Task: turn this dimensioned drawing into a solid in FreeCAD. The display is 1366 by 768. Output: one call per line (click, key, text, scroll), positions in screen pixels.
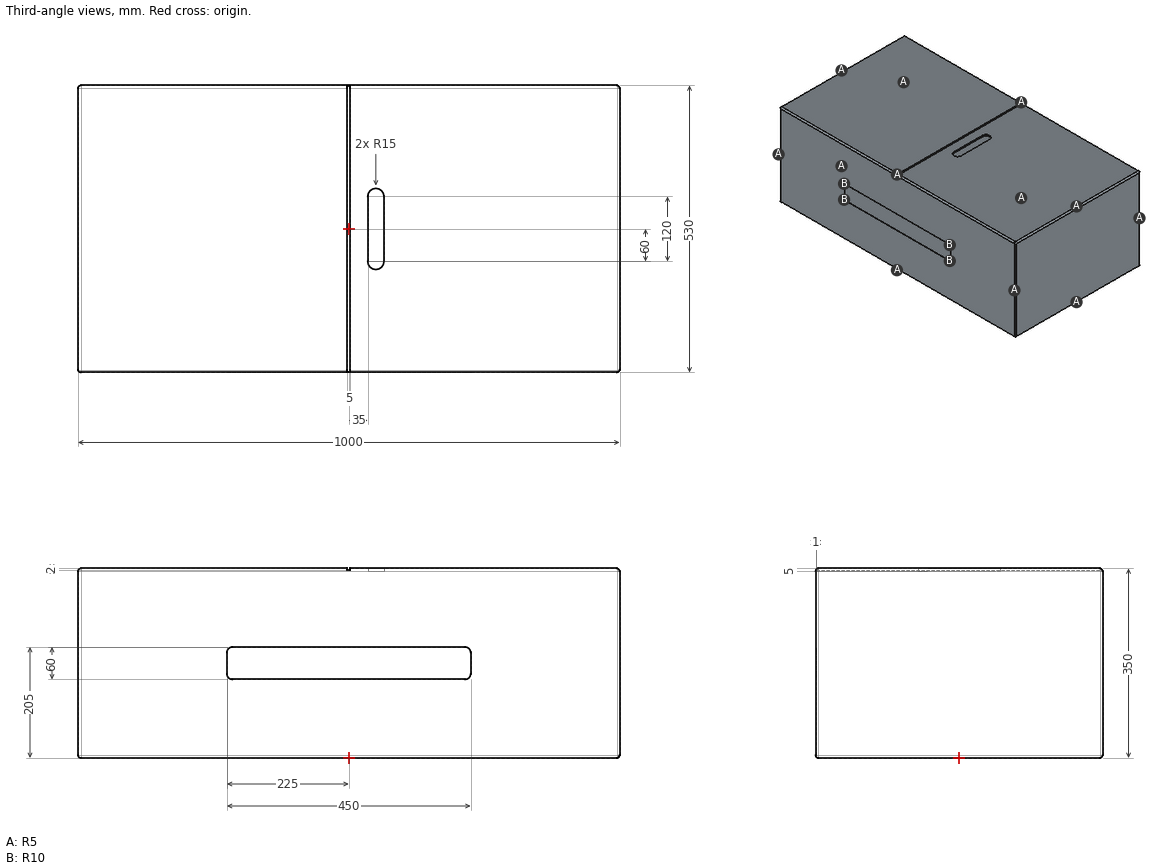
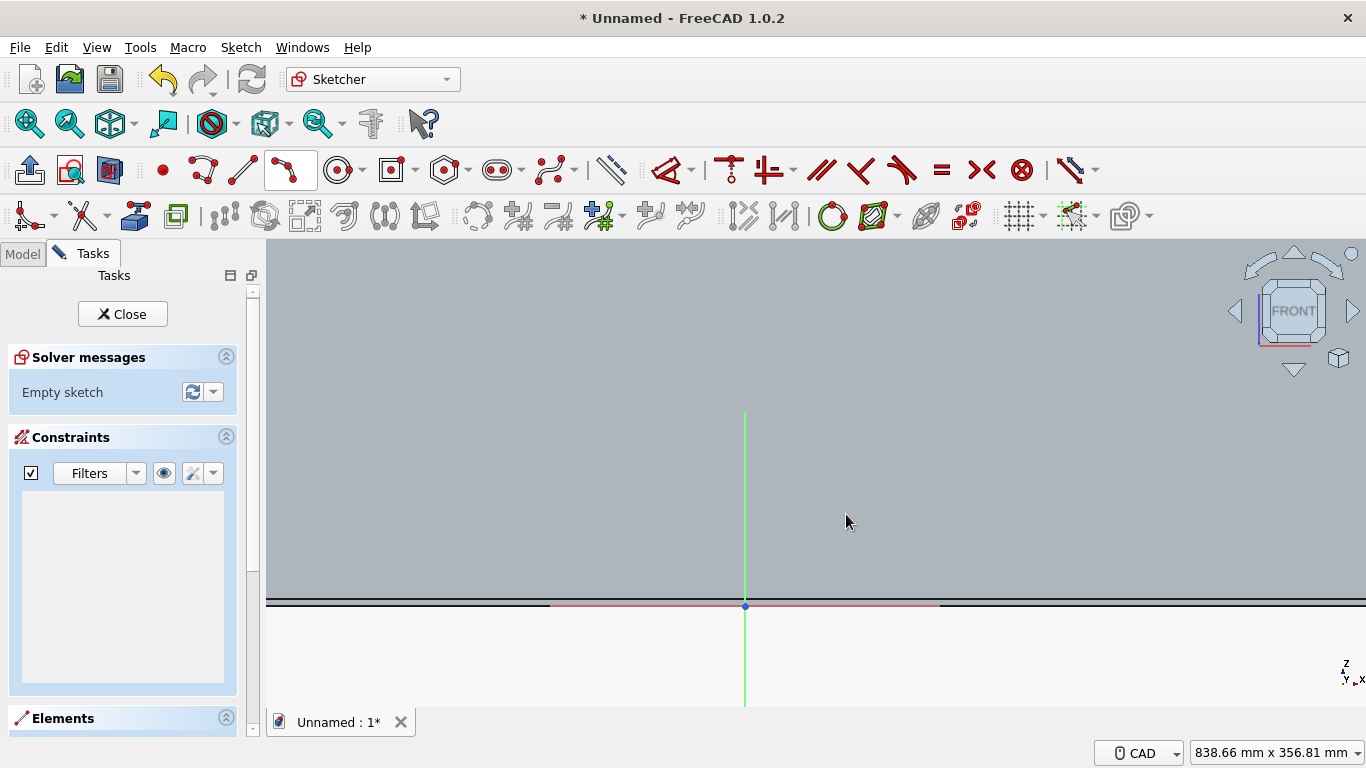
key(g)
key(r)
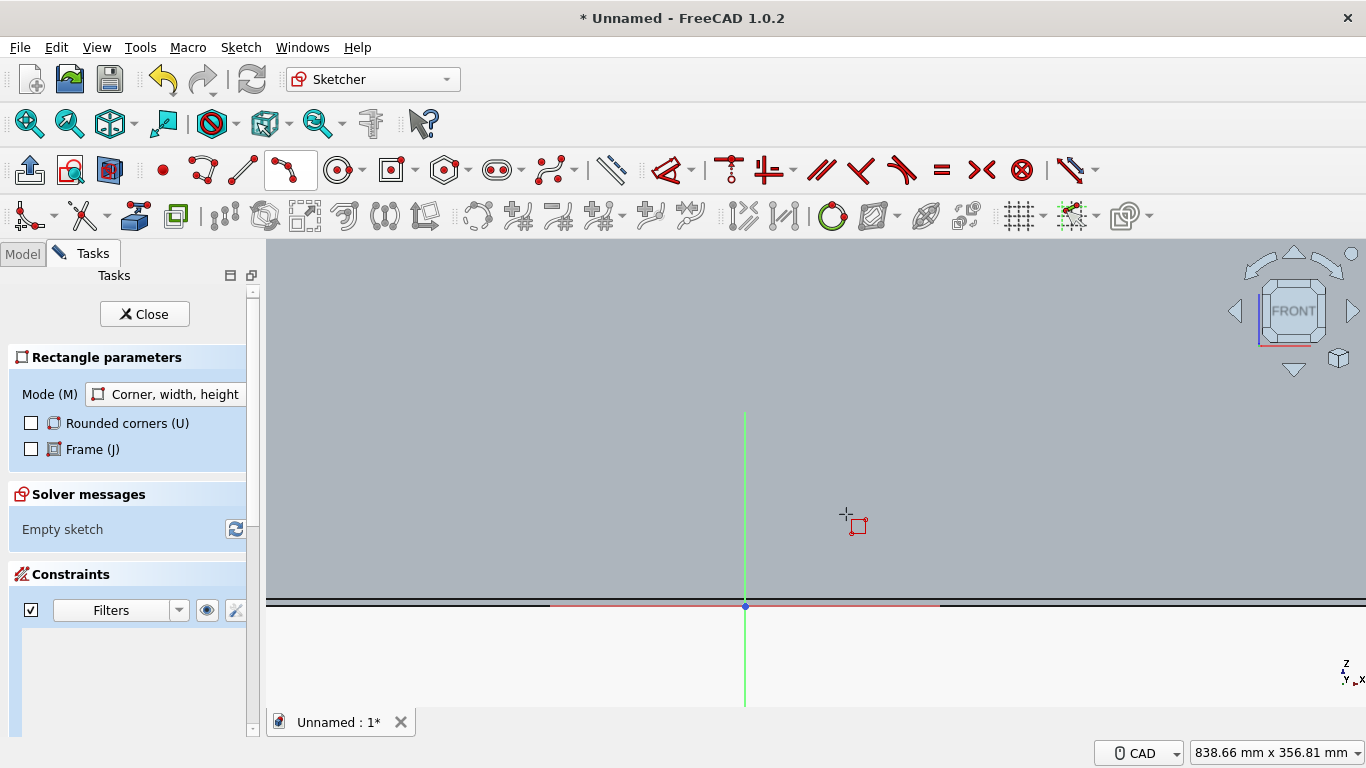
click(450, 337)
click(1040, 416)
key(Escape)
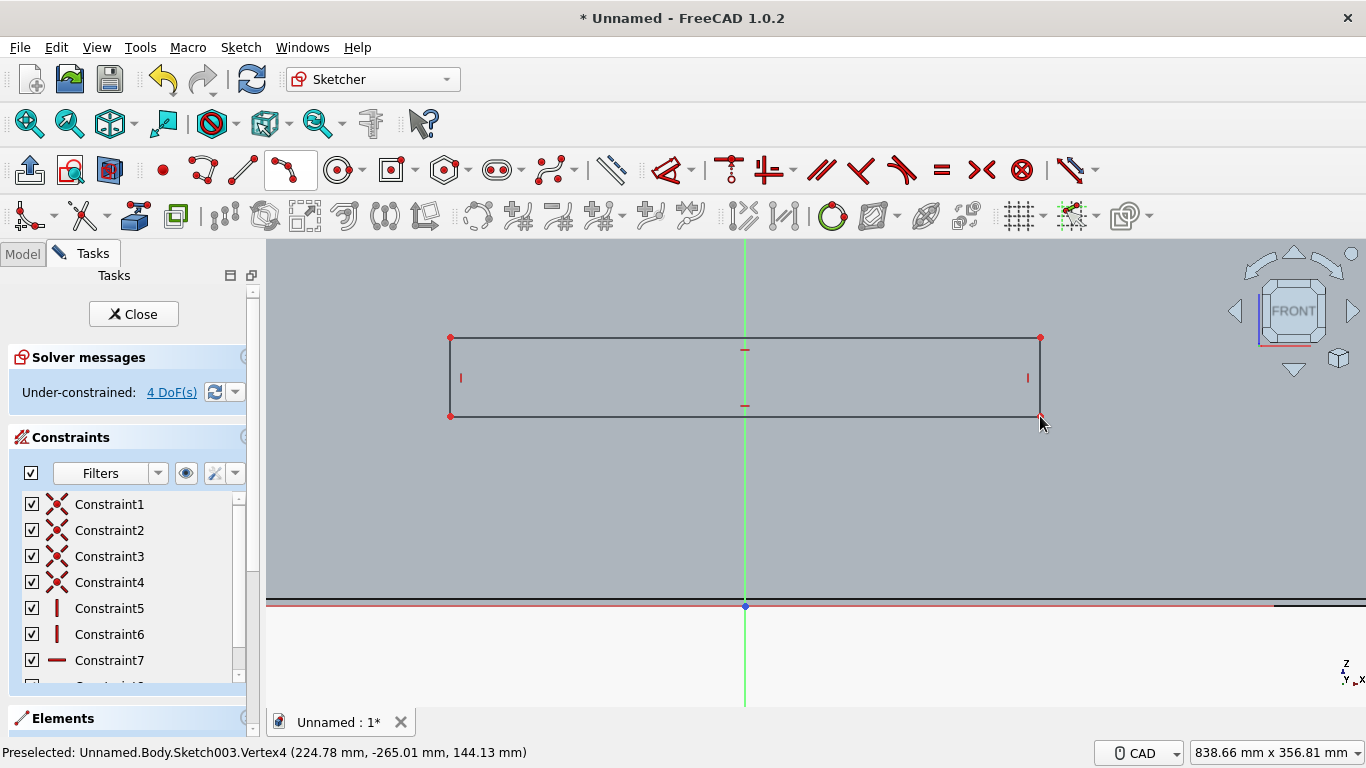
click(666, 170)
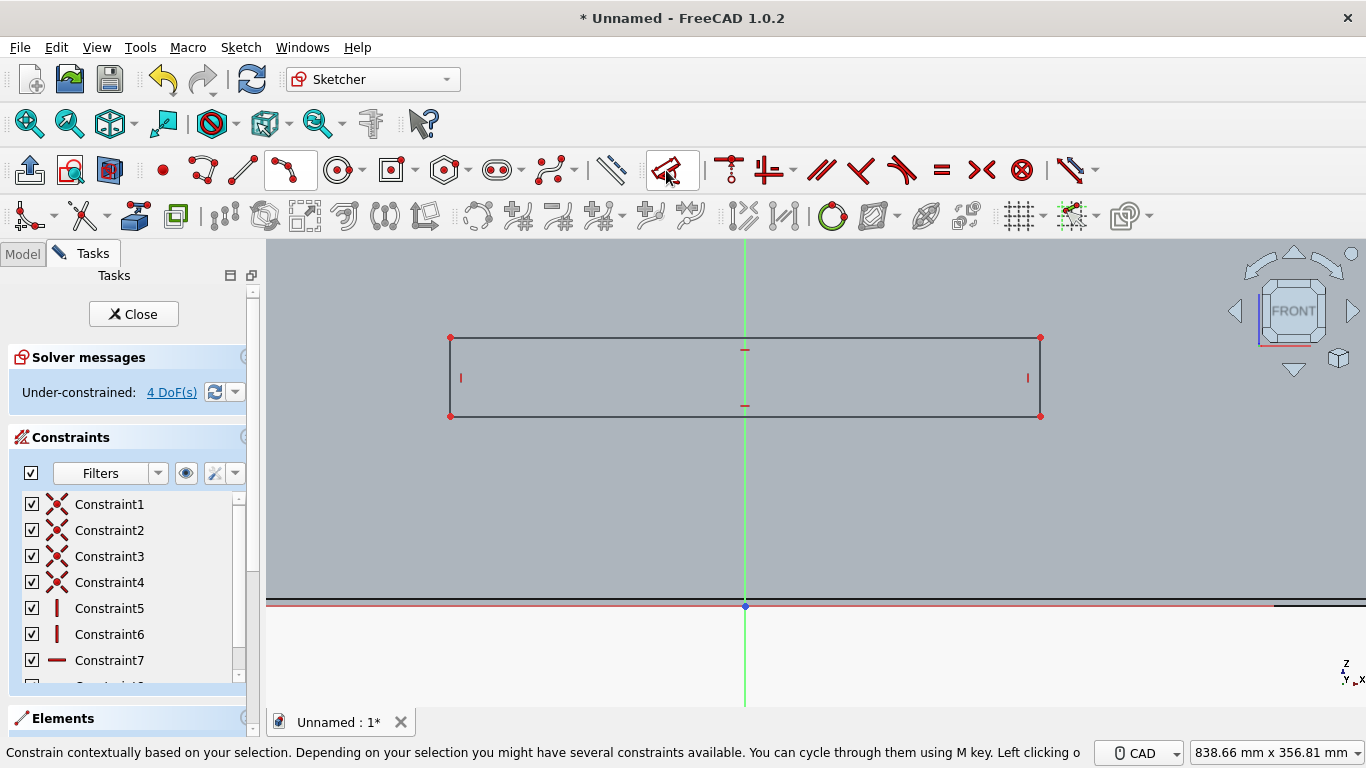
click(450, 362)
click(416, 378)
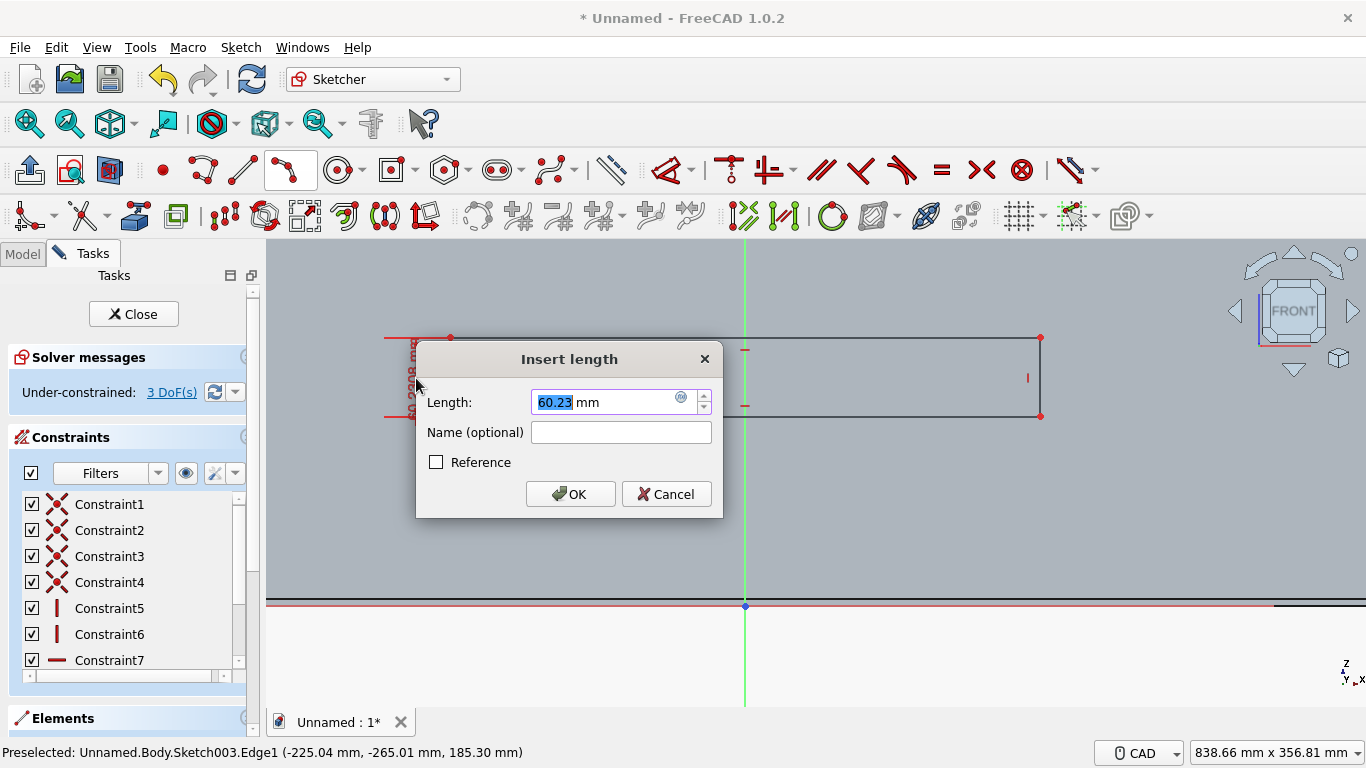
text(60)
key(Return)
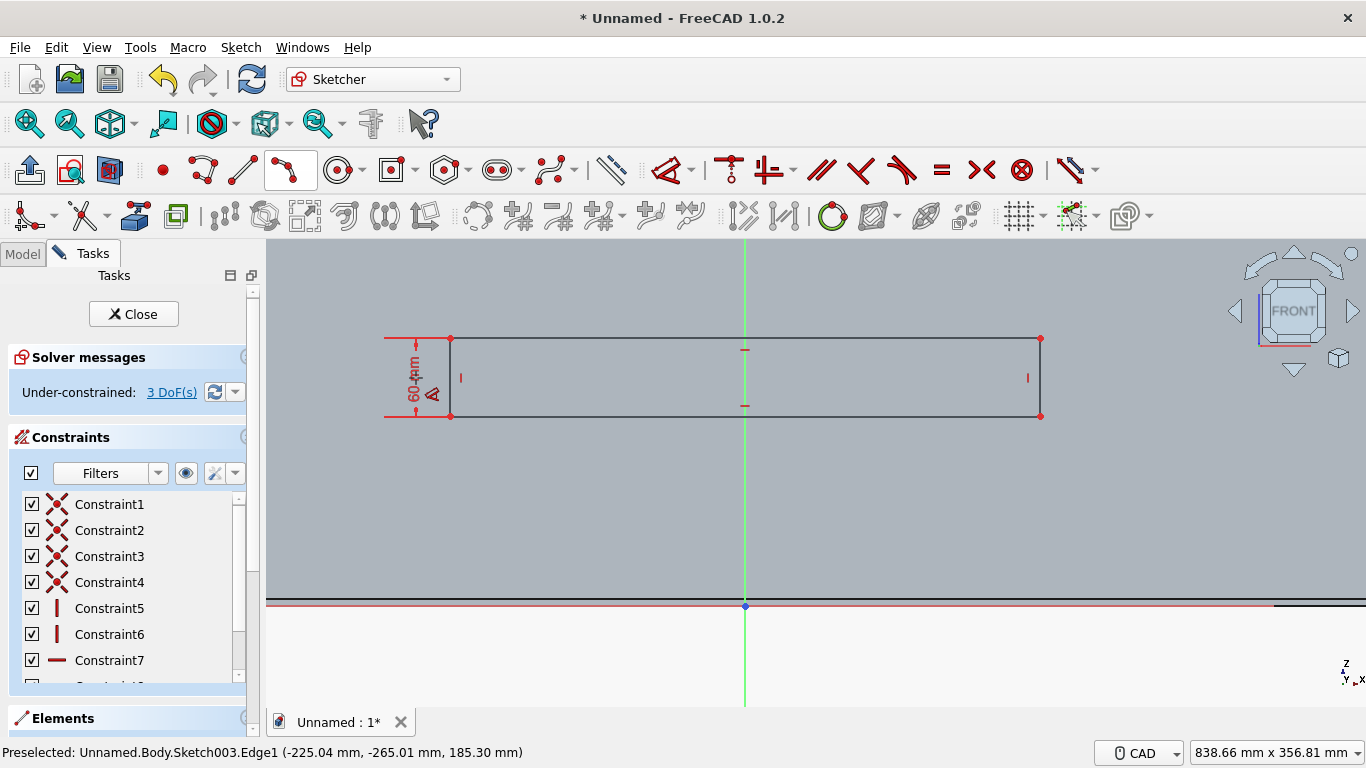
click(627, 417)
click(609, 383)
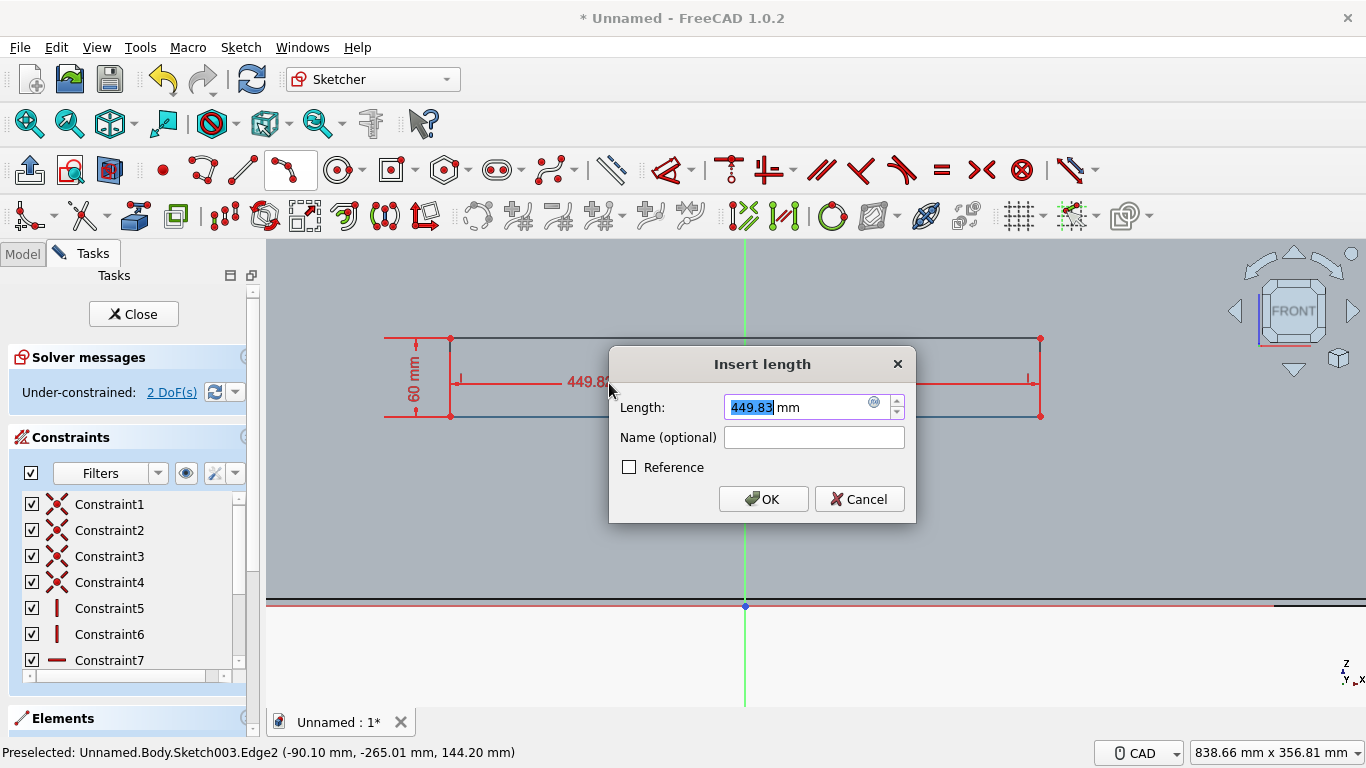
text(450)
key(Return)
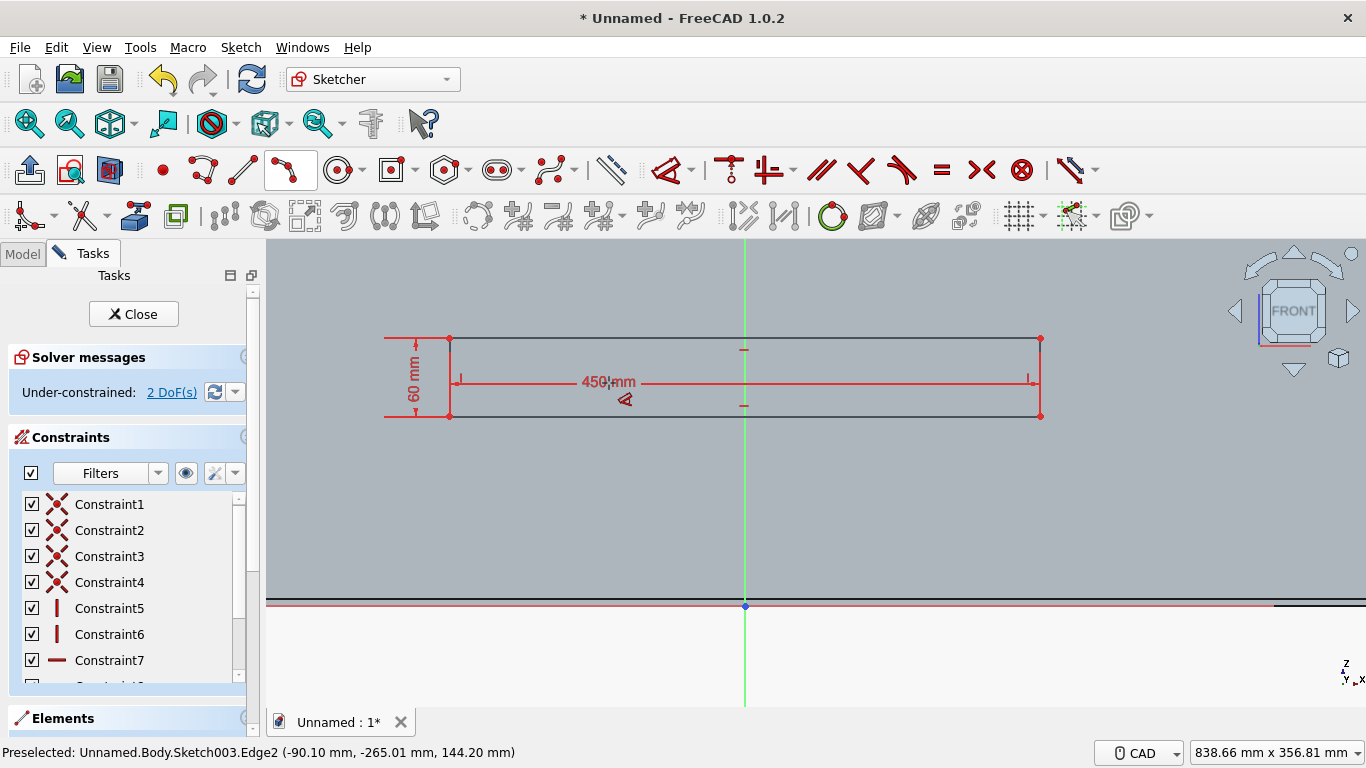
click(450, 338)
click(598, 640)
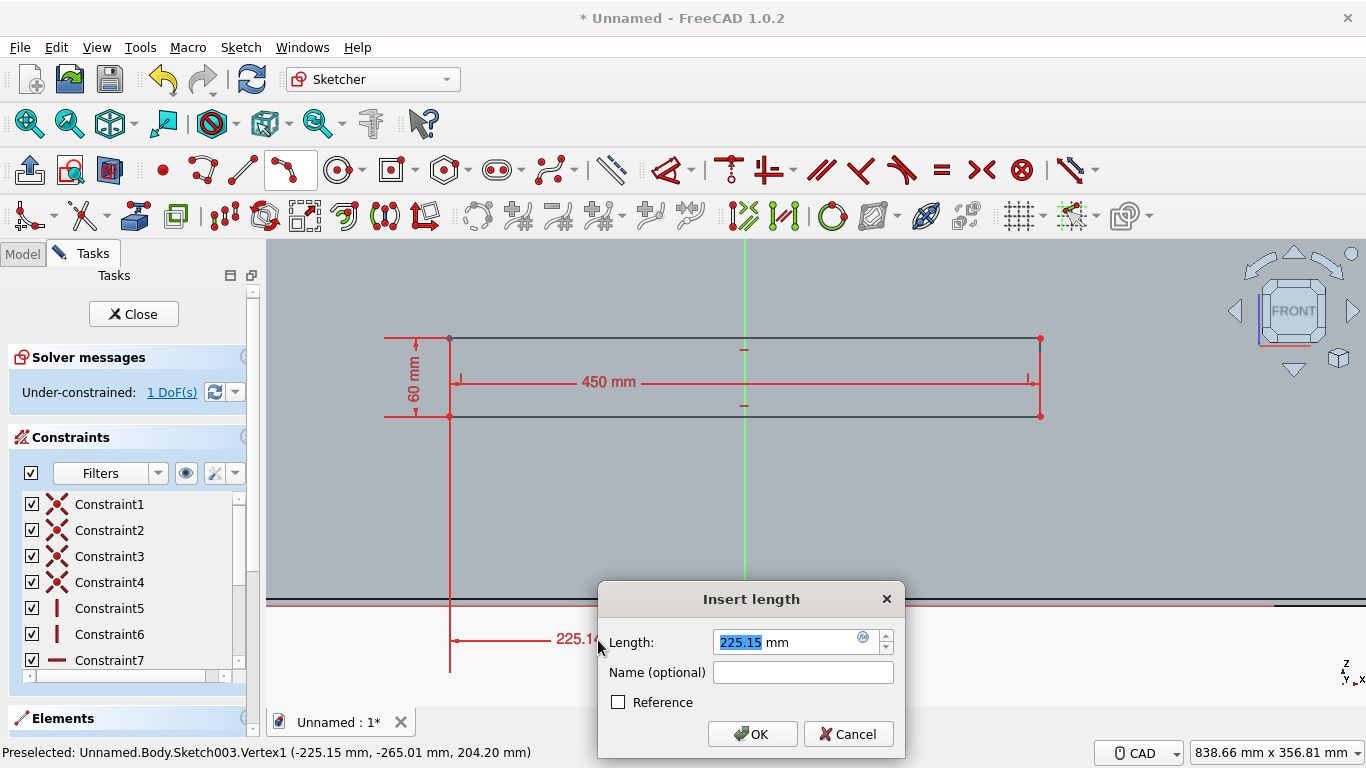
text(225)
key(Return)